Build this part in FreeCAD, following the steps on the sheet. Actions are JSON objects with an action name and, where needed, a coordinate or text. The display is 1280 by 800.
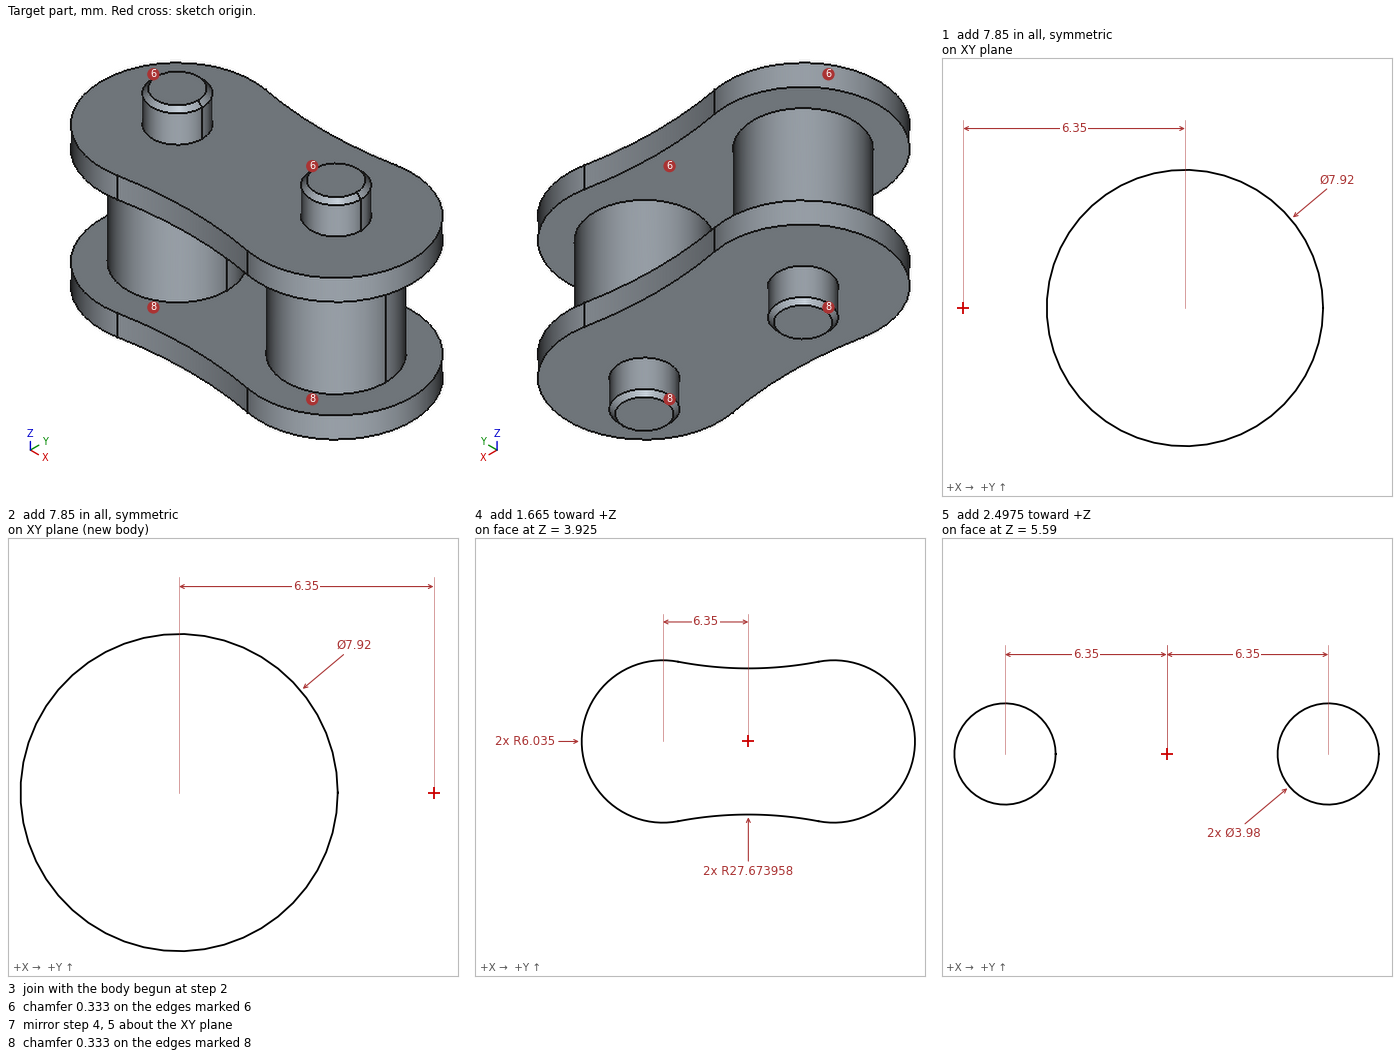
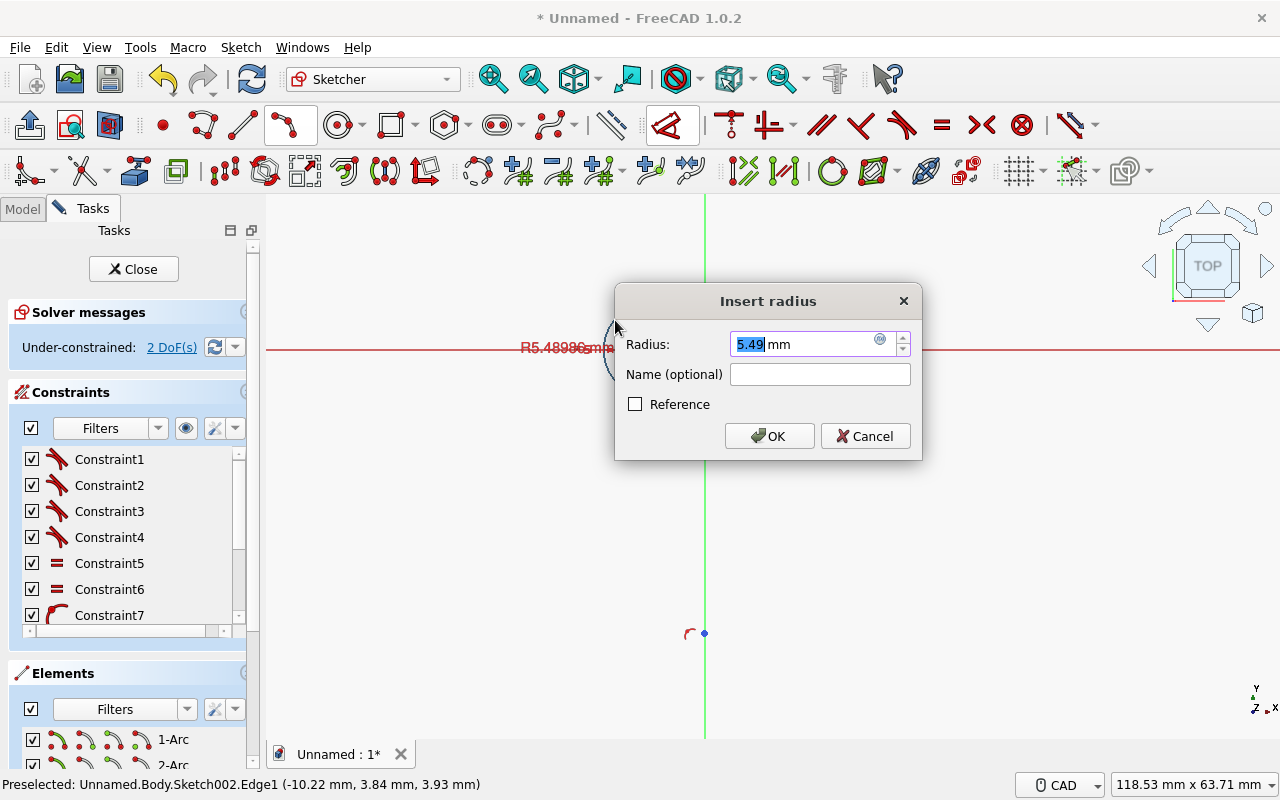
{"action": "type", "text": "6.035"}
{"action": "key", "text": "Return"}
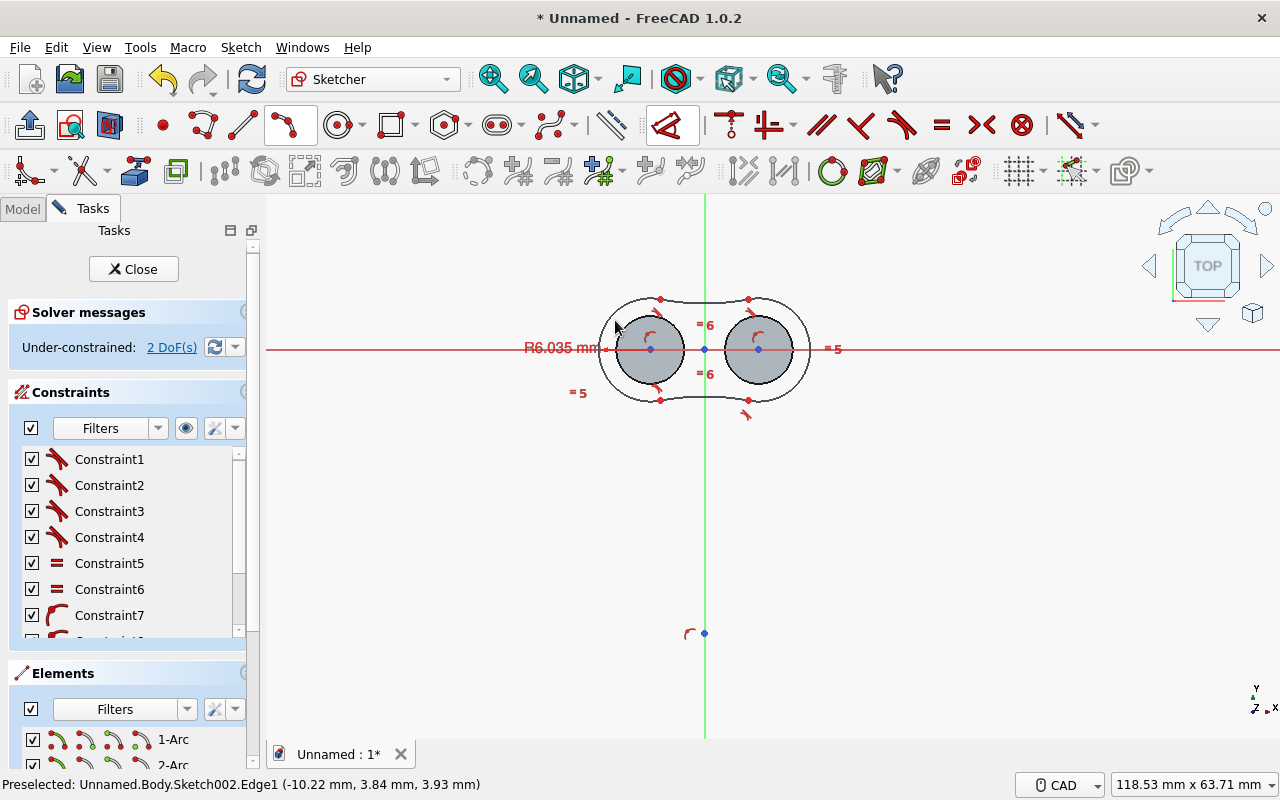
{"action": "left_click", "coordinate": [722, 397]}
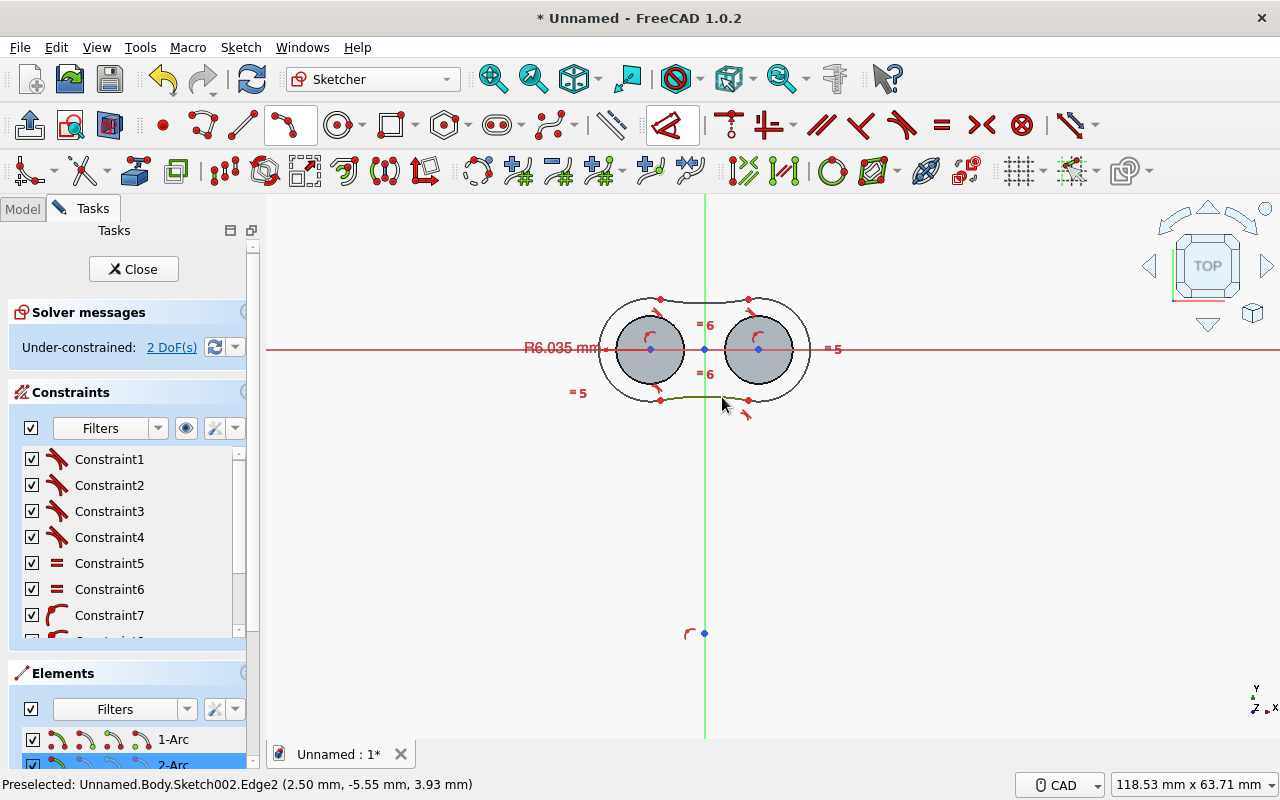
{"action": "left_click", "coordinate": [694, 126]}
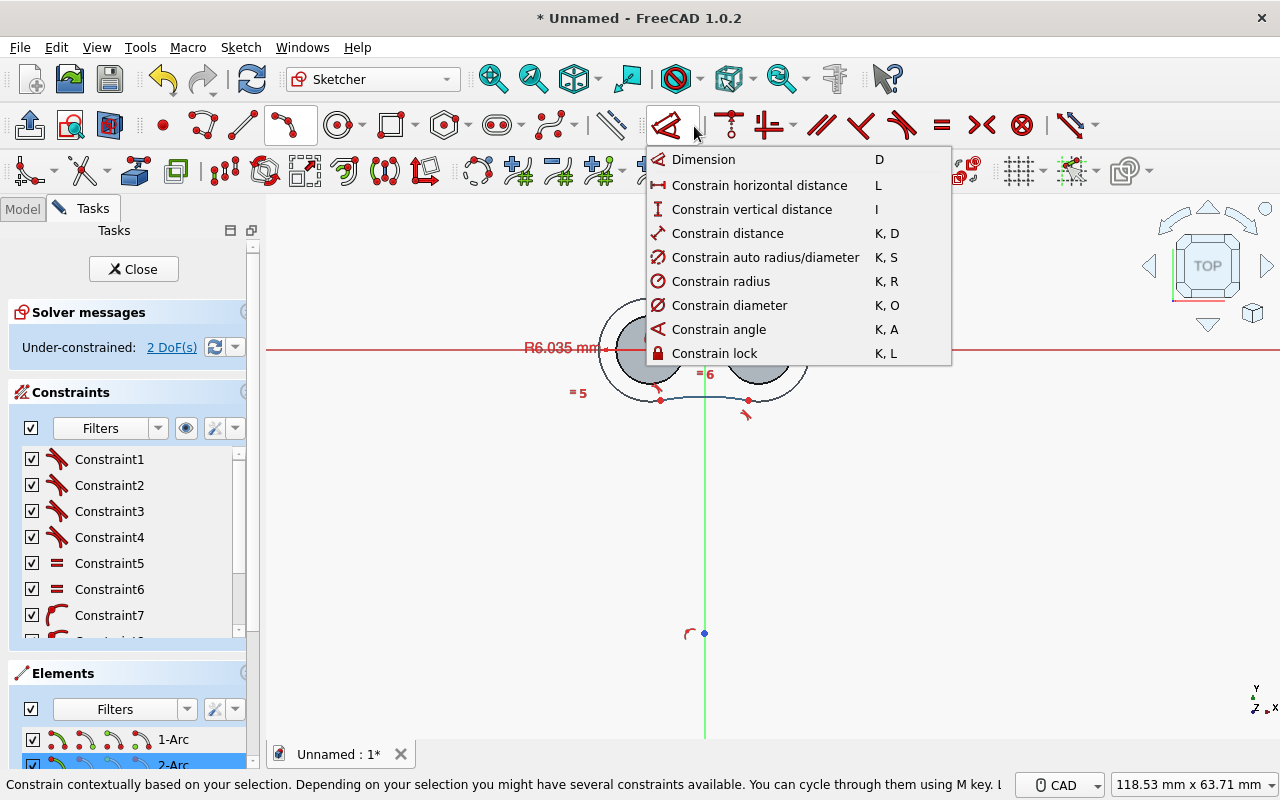
{"action": "left_click", "coordinate": [799, 281]}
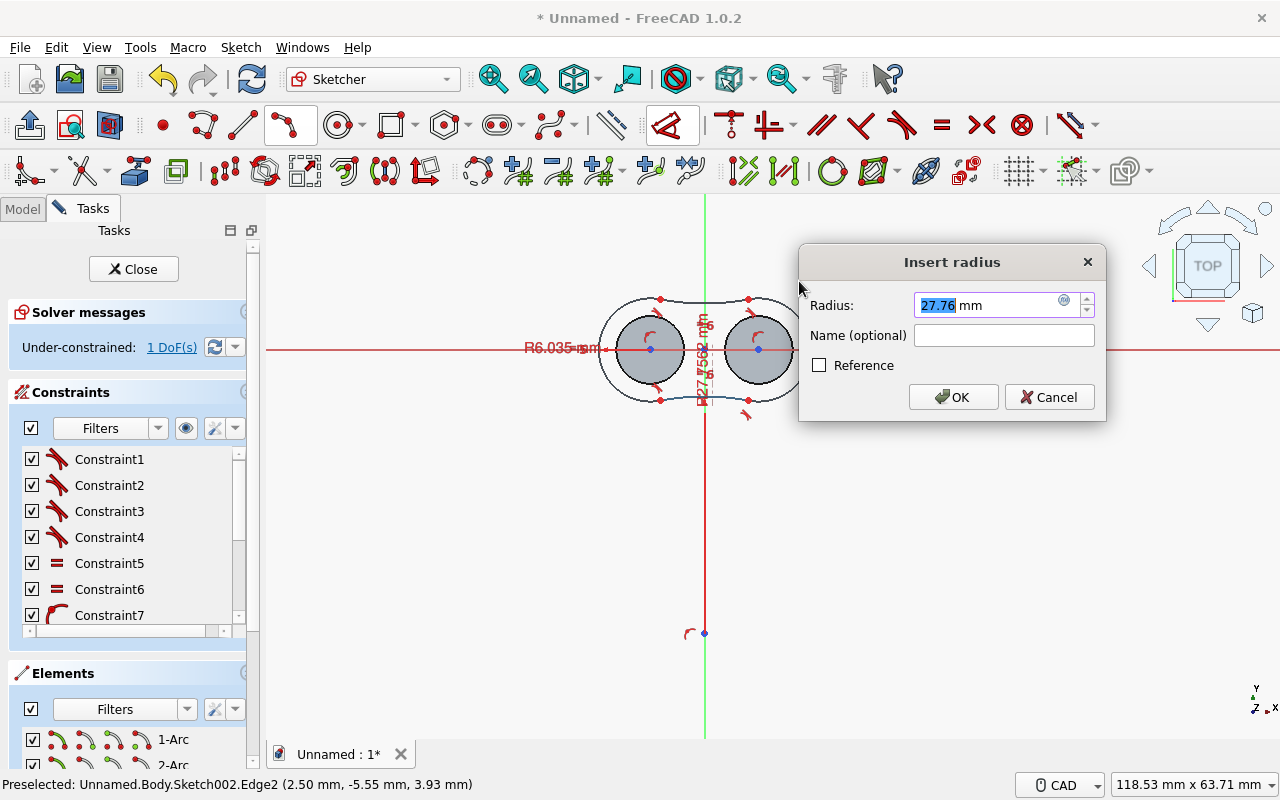
{"action": "type", "text": "27.673958"}
{"action": "key", "text": "Return"}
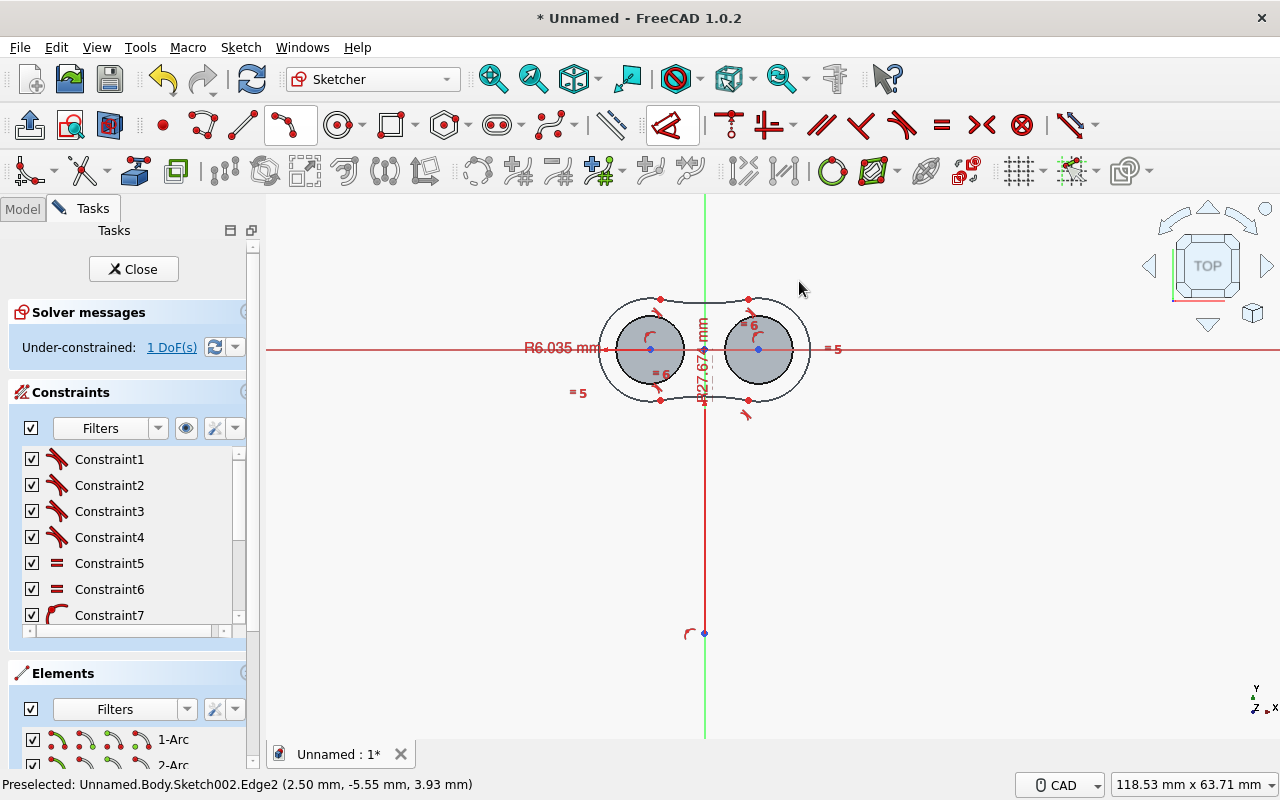
{"action": "left_click", "coordinate": [650, 350]}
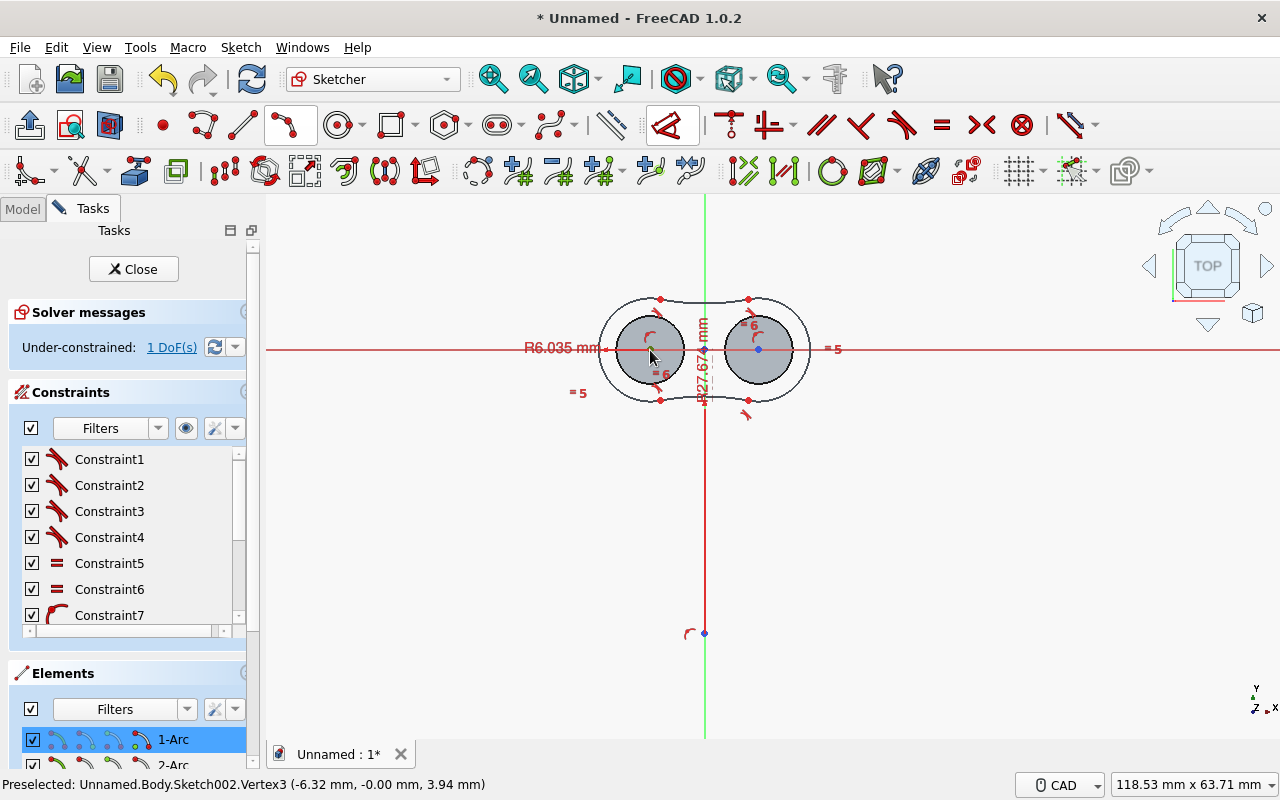
{"action": "left_click", "coordinate": [694, 126]}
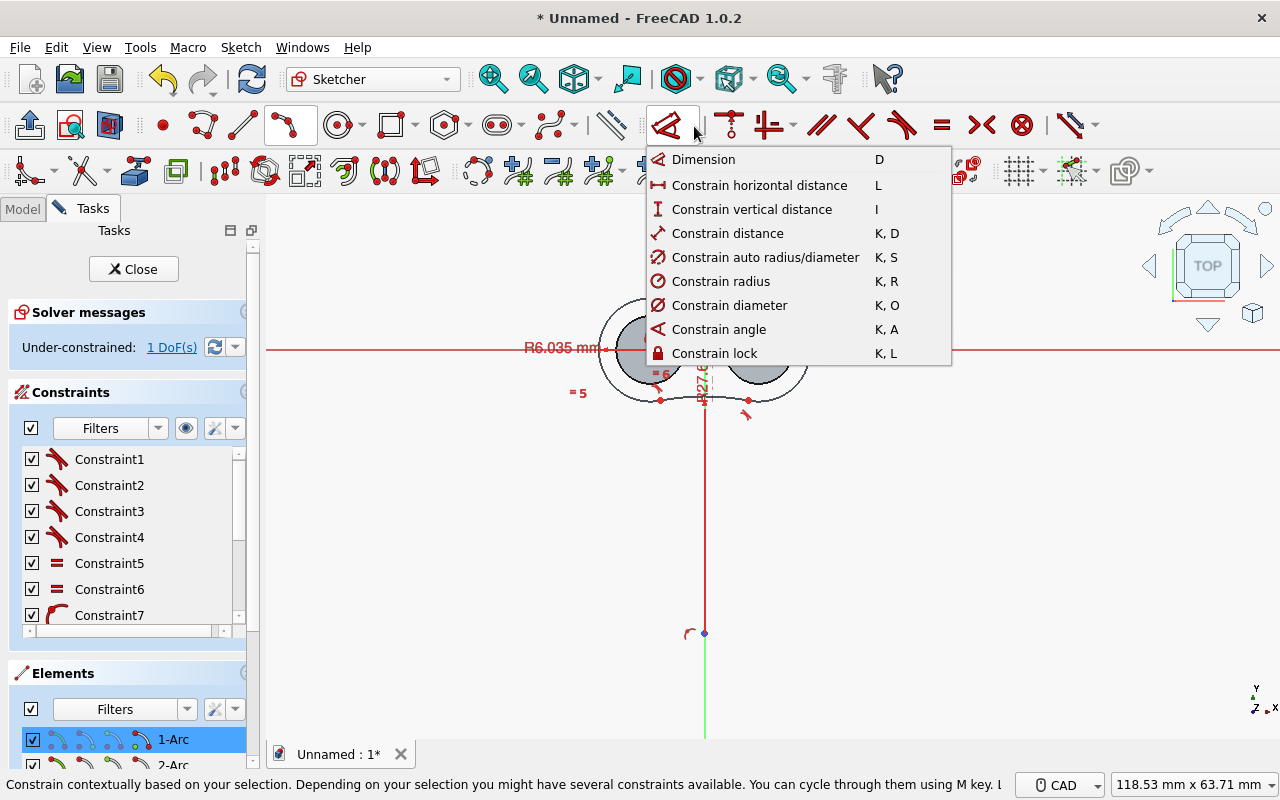
{"action": "left_click", "coordinate": [799, 185]}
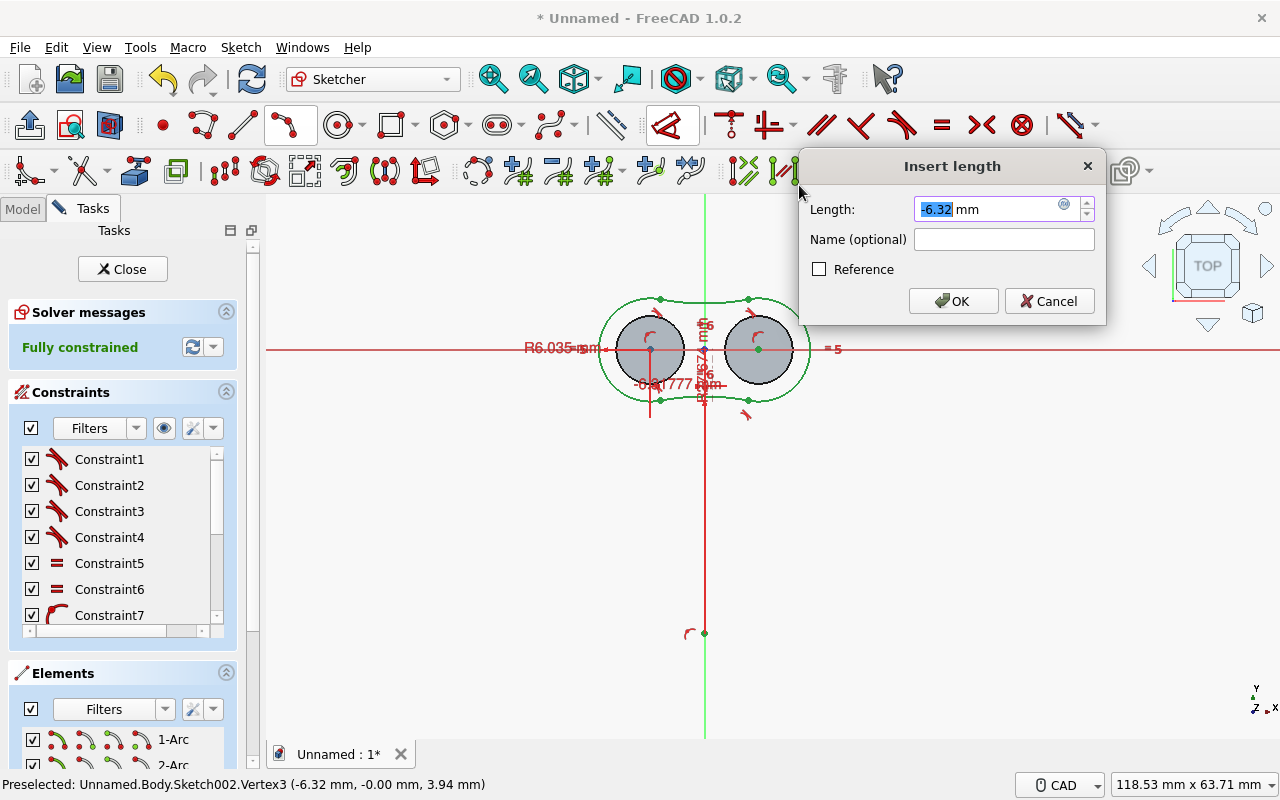
{"action": "type", "text": "-6.35"}
{"action": "key", "text": "Return"}